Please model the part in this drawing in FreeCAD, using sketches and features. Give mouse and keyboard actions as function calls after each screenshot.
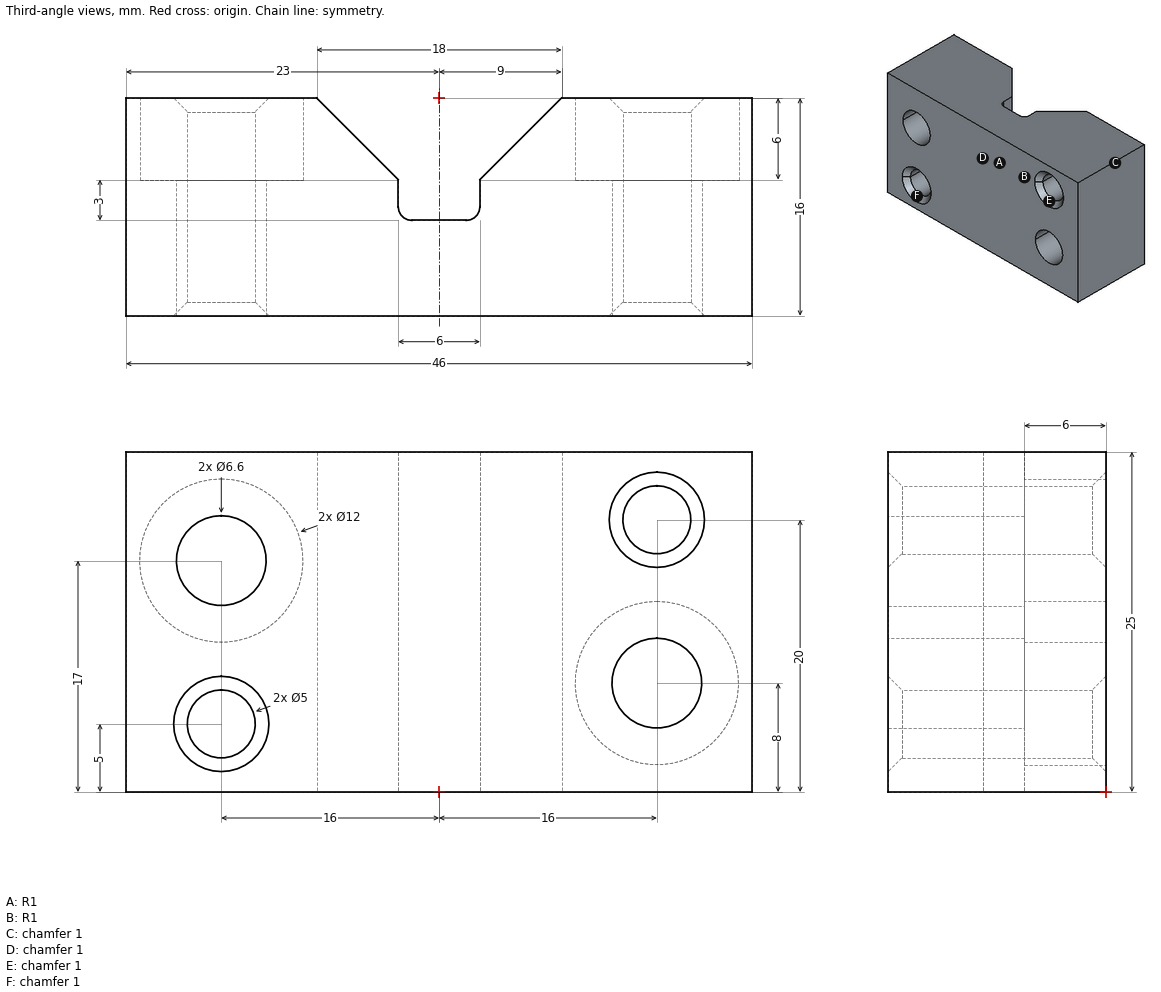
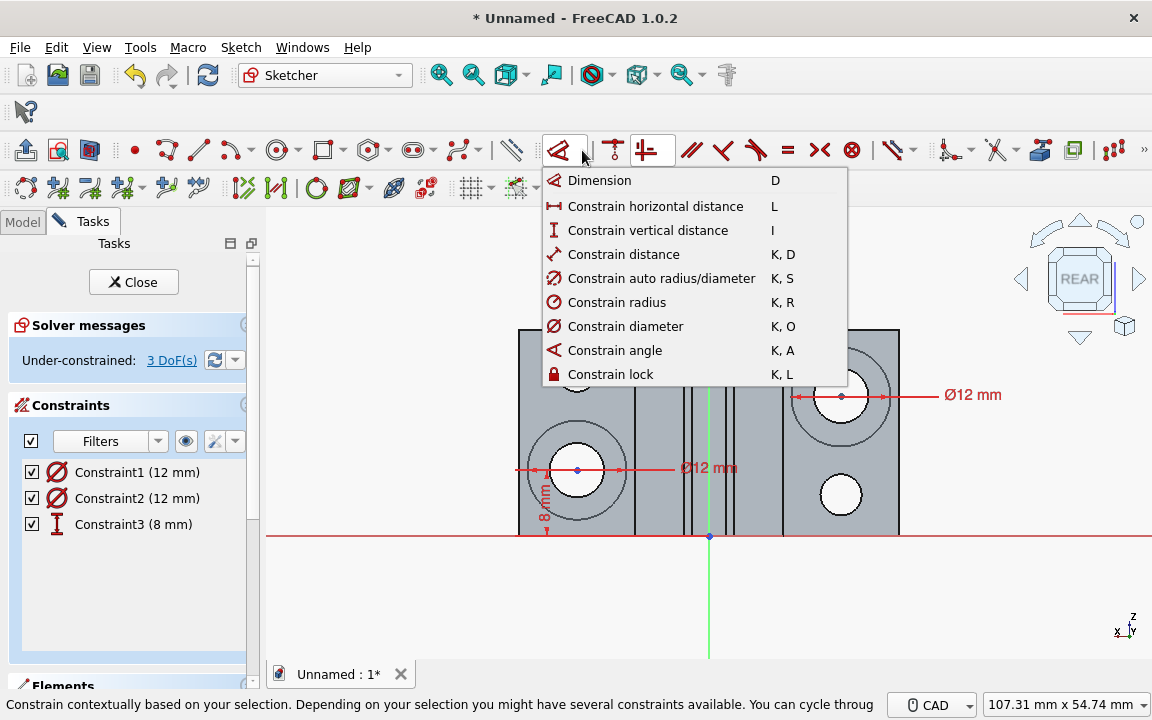
click(695, 206)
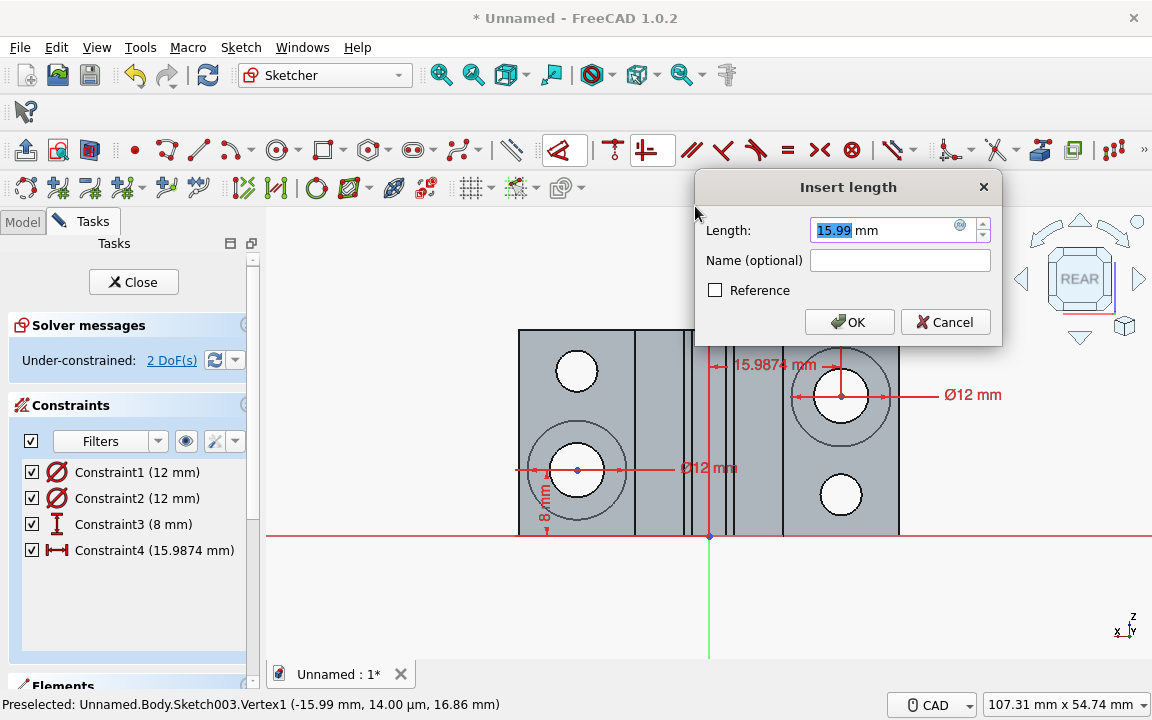
text(16)
key(Return)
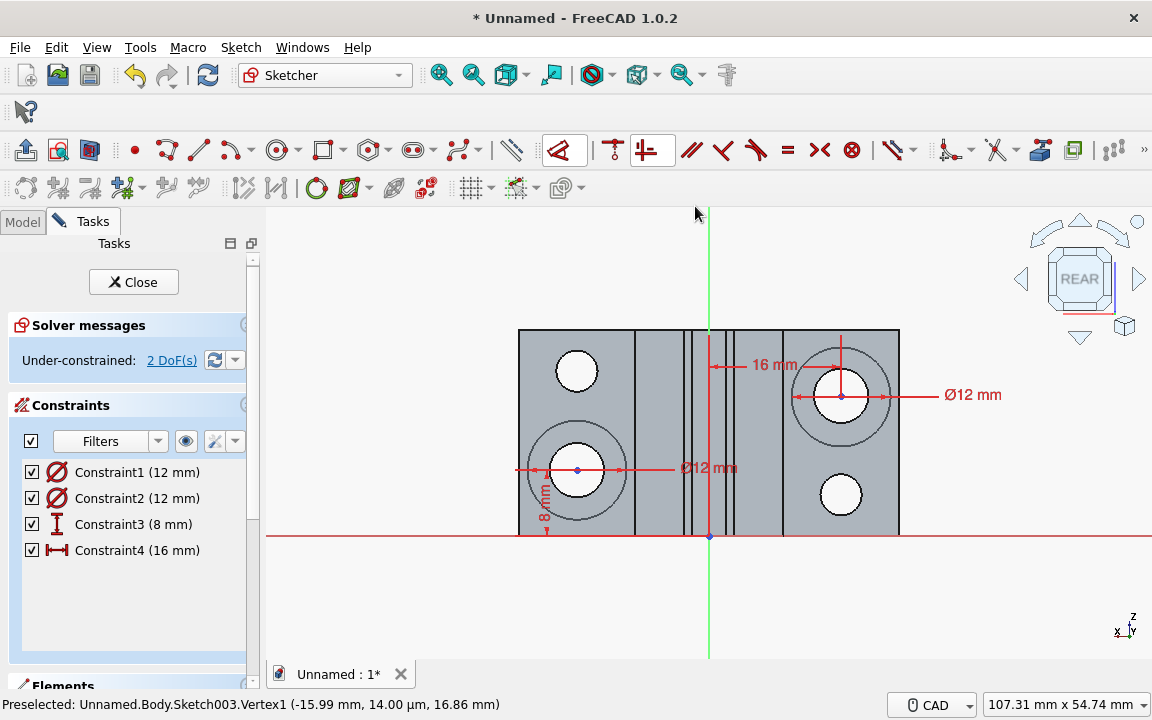
click(841, 397)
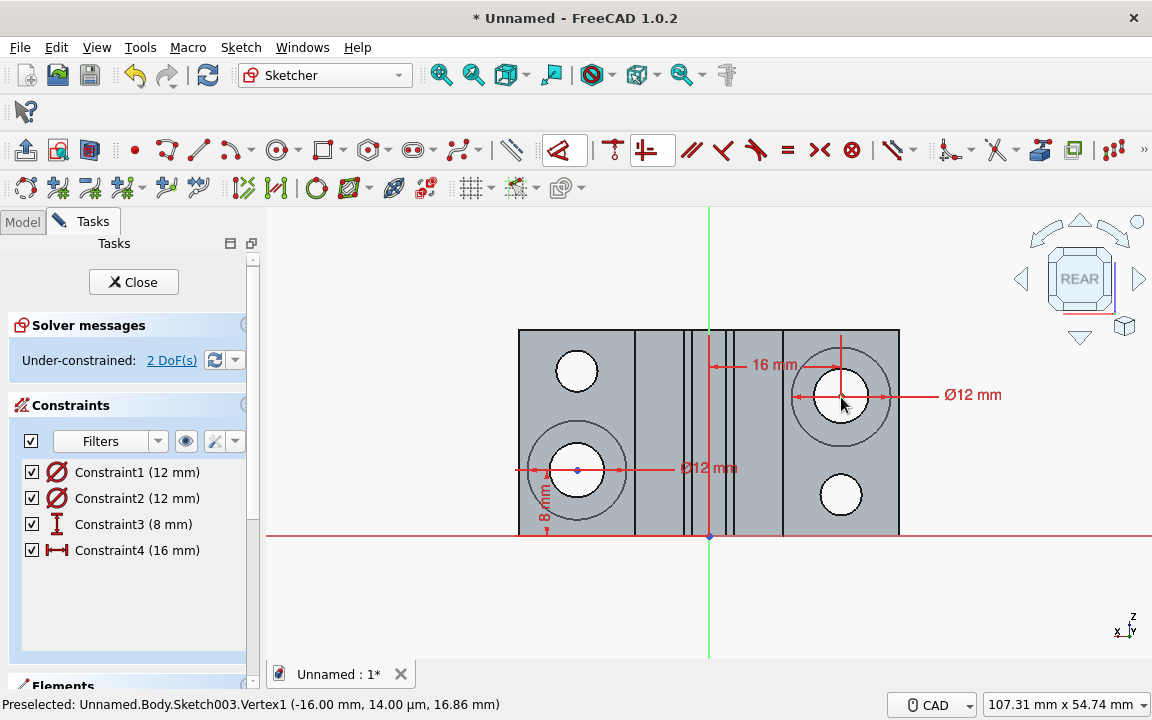
click(582, 150)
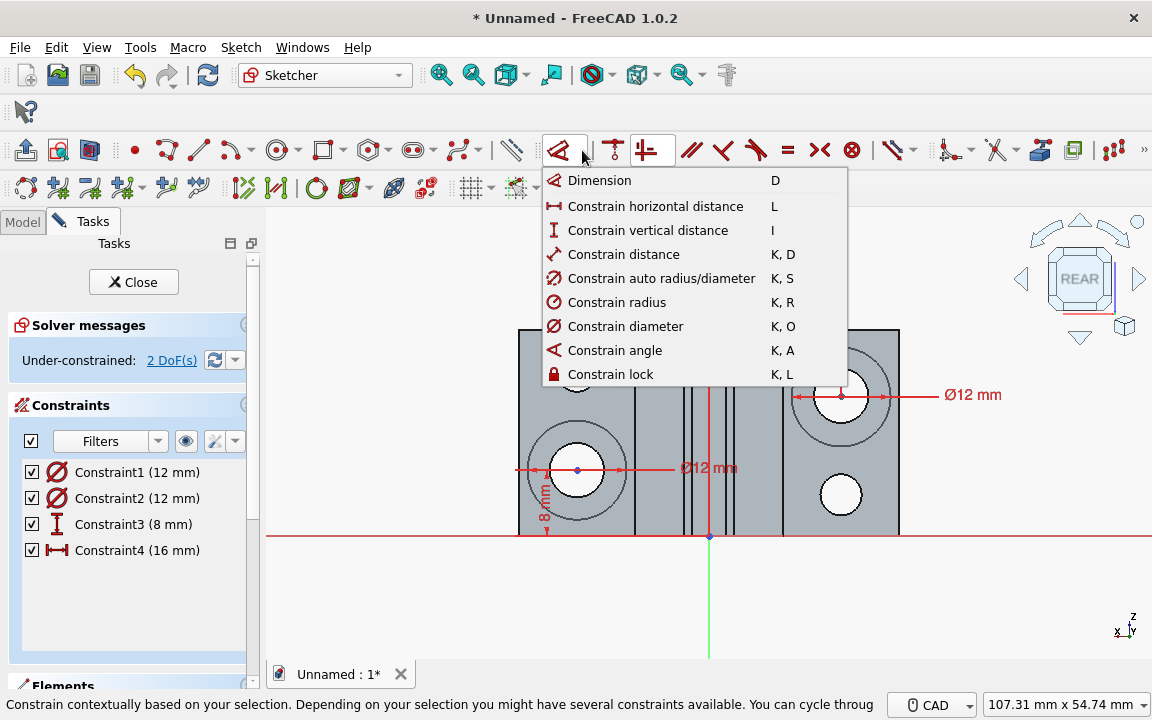
click(695, 230)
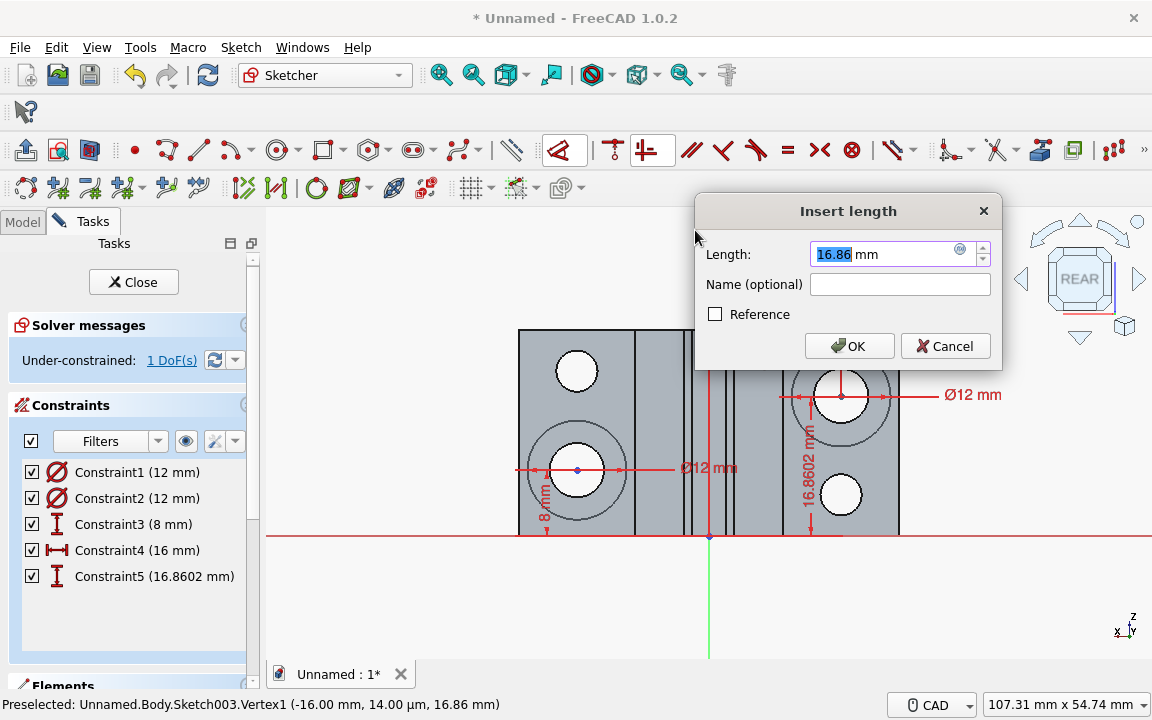
text(17)
key(Return)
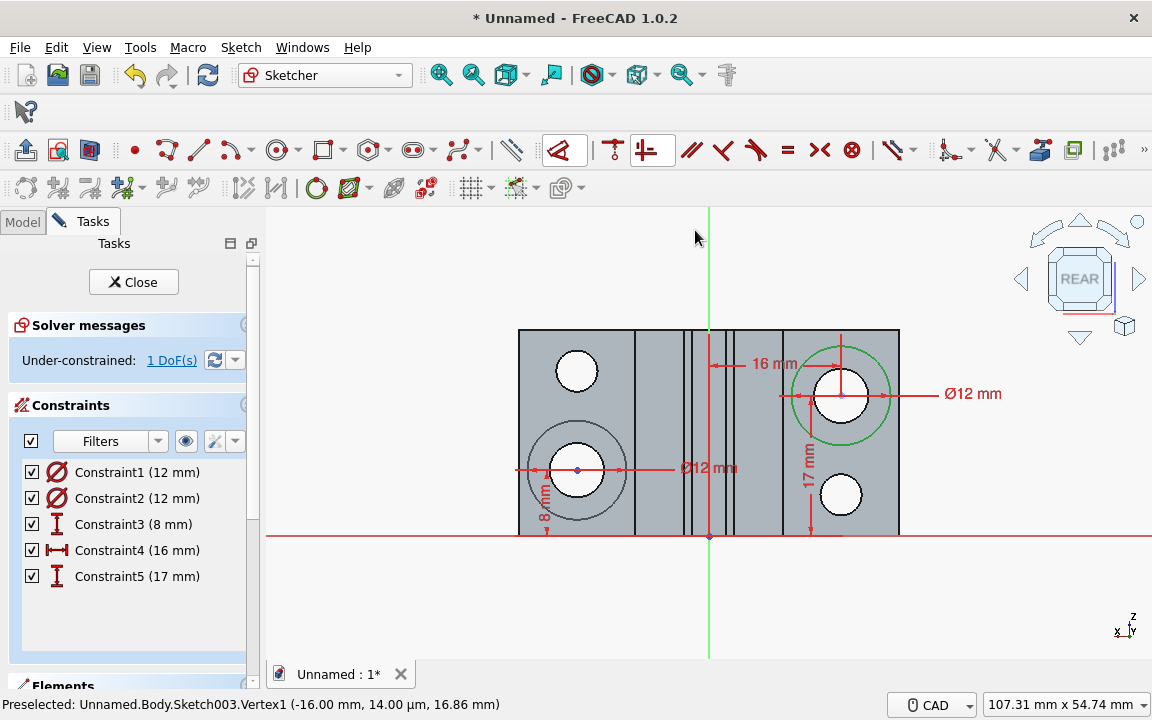
click(577, 470)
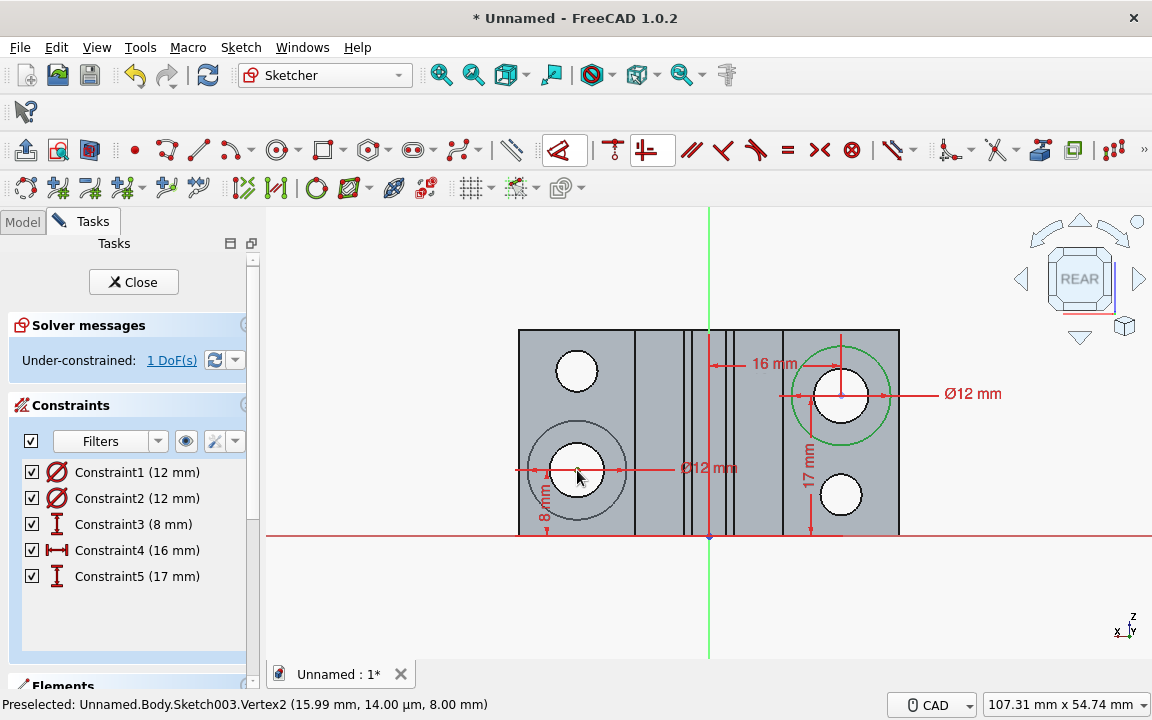
click(582, 150)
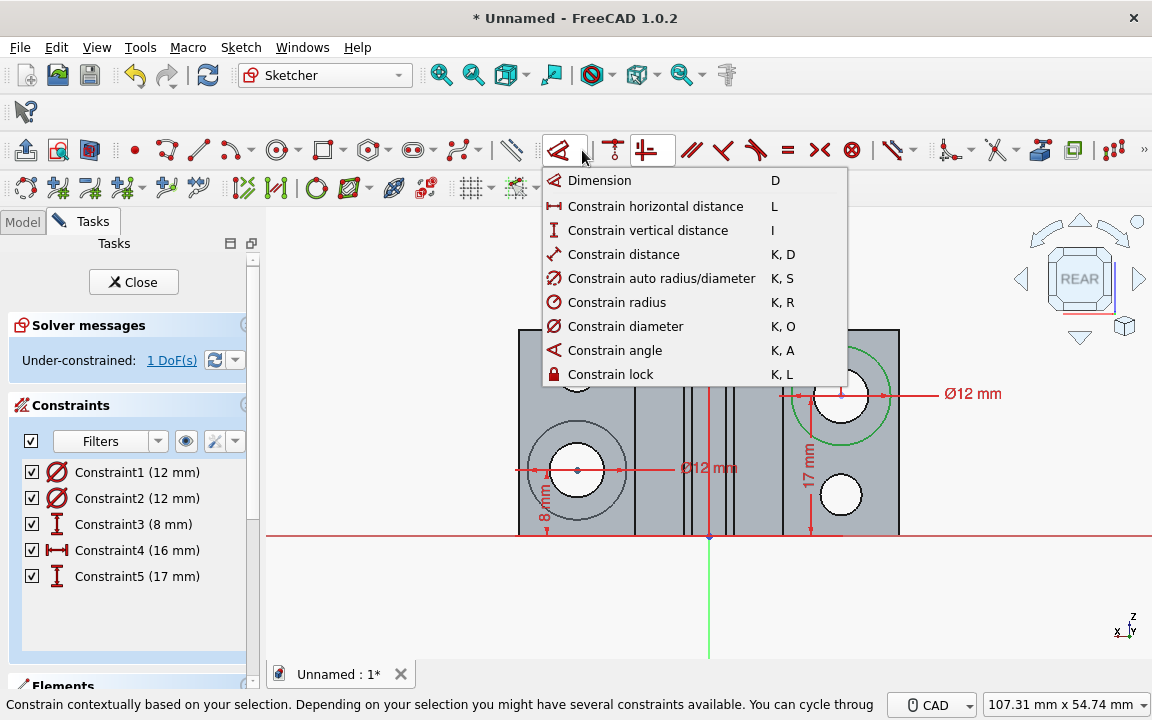
click(695, 206)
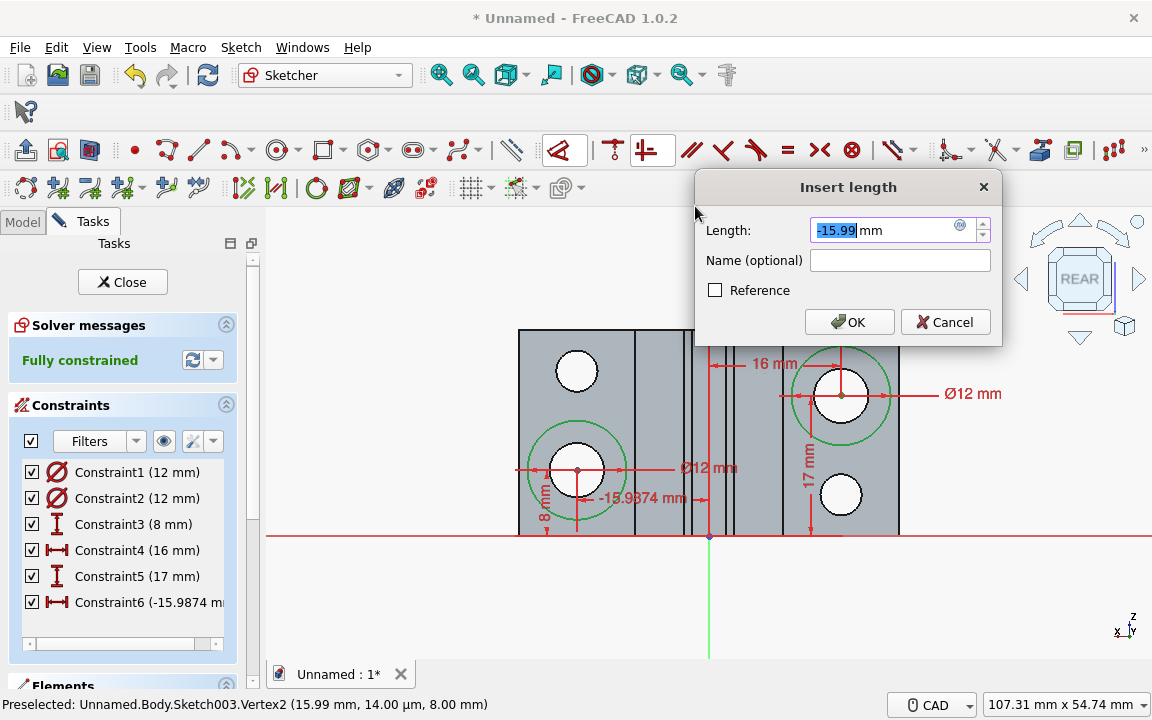
text(-16)
key(Return)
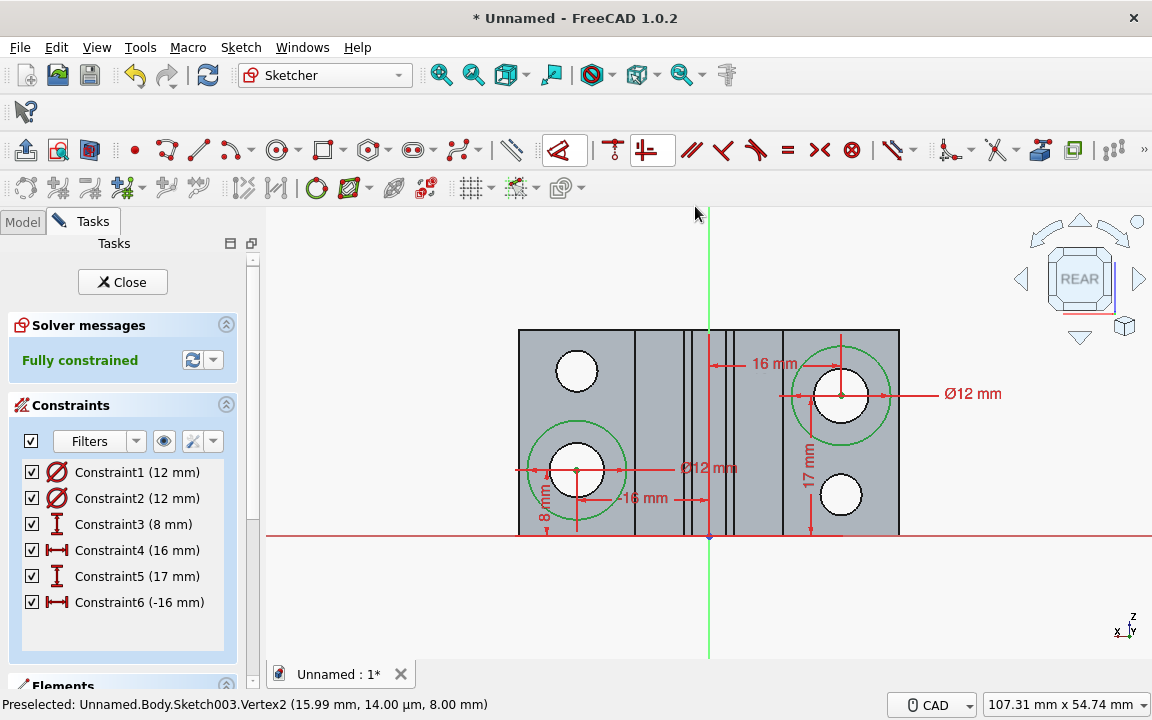
click(123, 282)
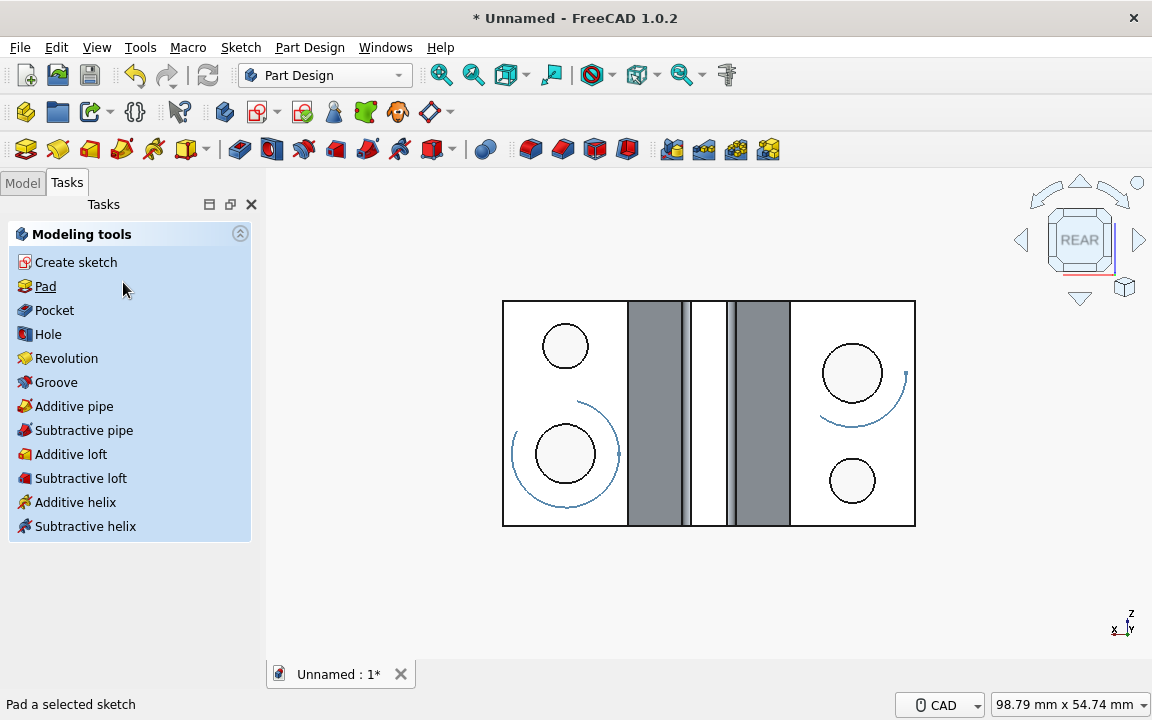
click(240, 150)